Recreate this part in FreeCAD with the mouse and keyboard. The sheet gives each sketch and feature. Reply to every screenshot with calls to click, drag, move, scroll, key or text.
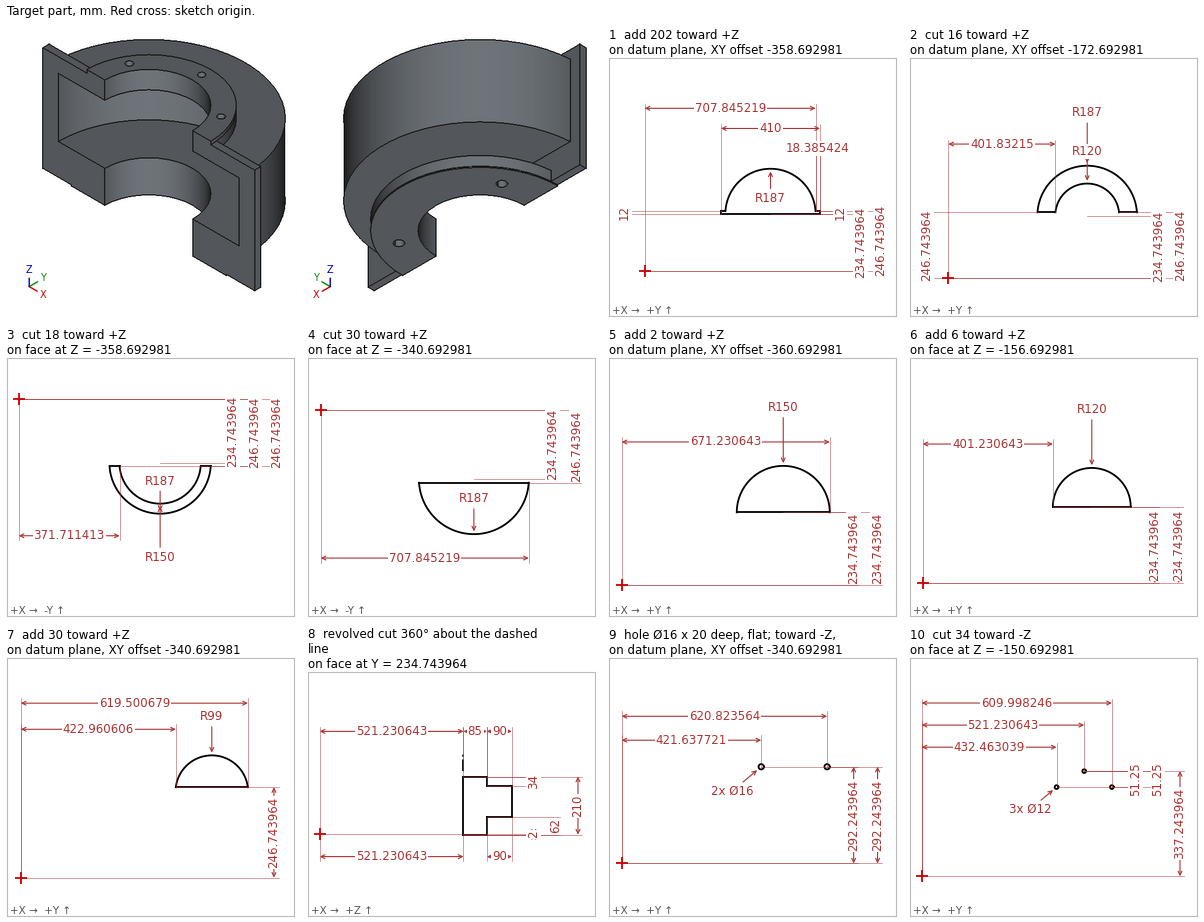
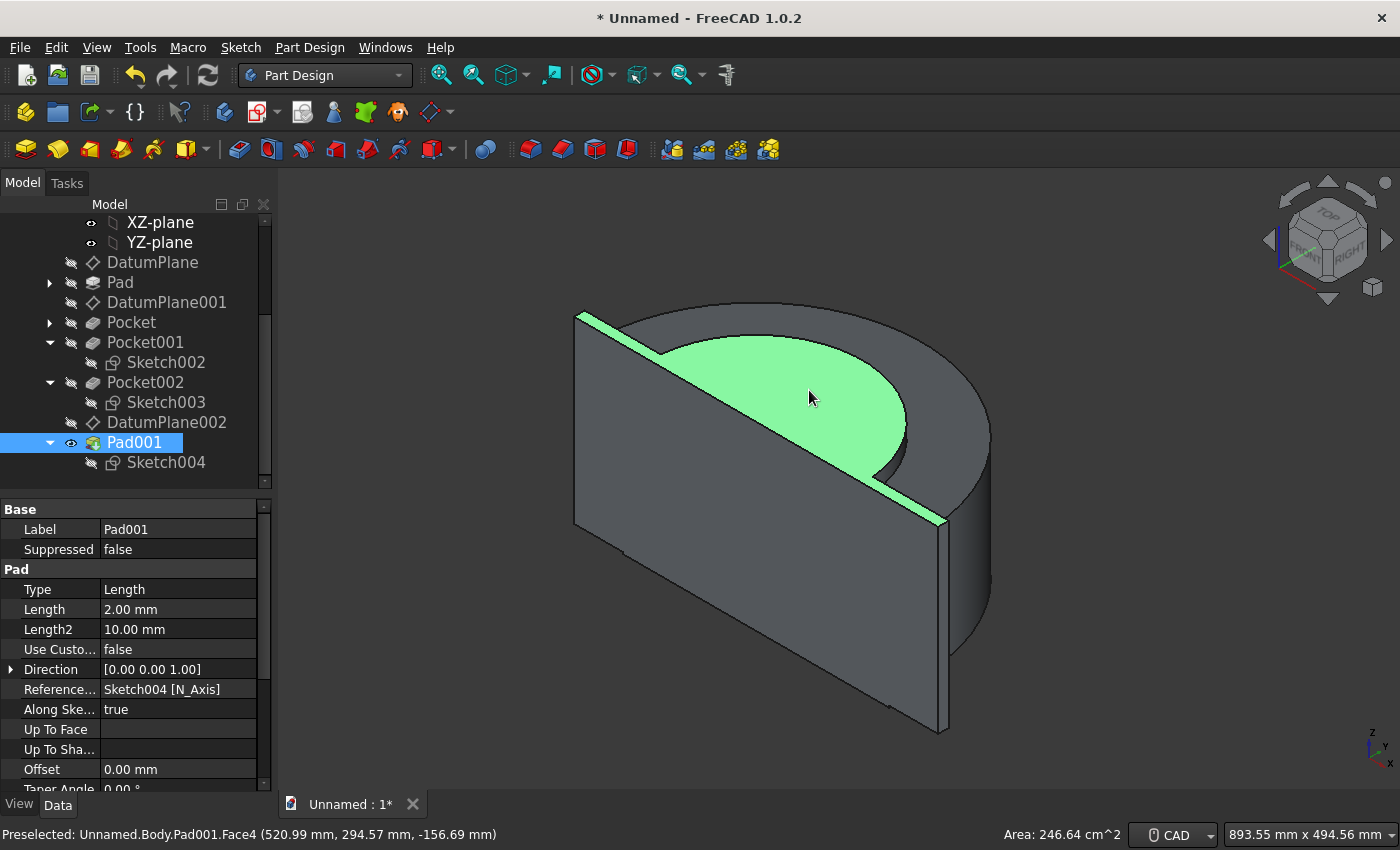
click(258, 112)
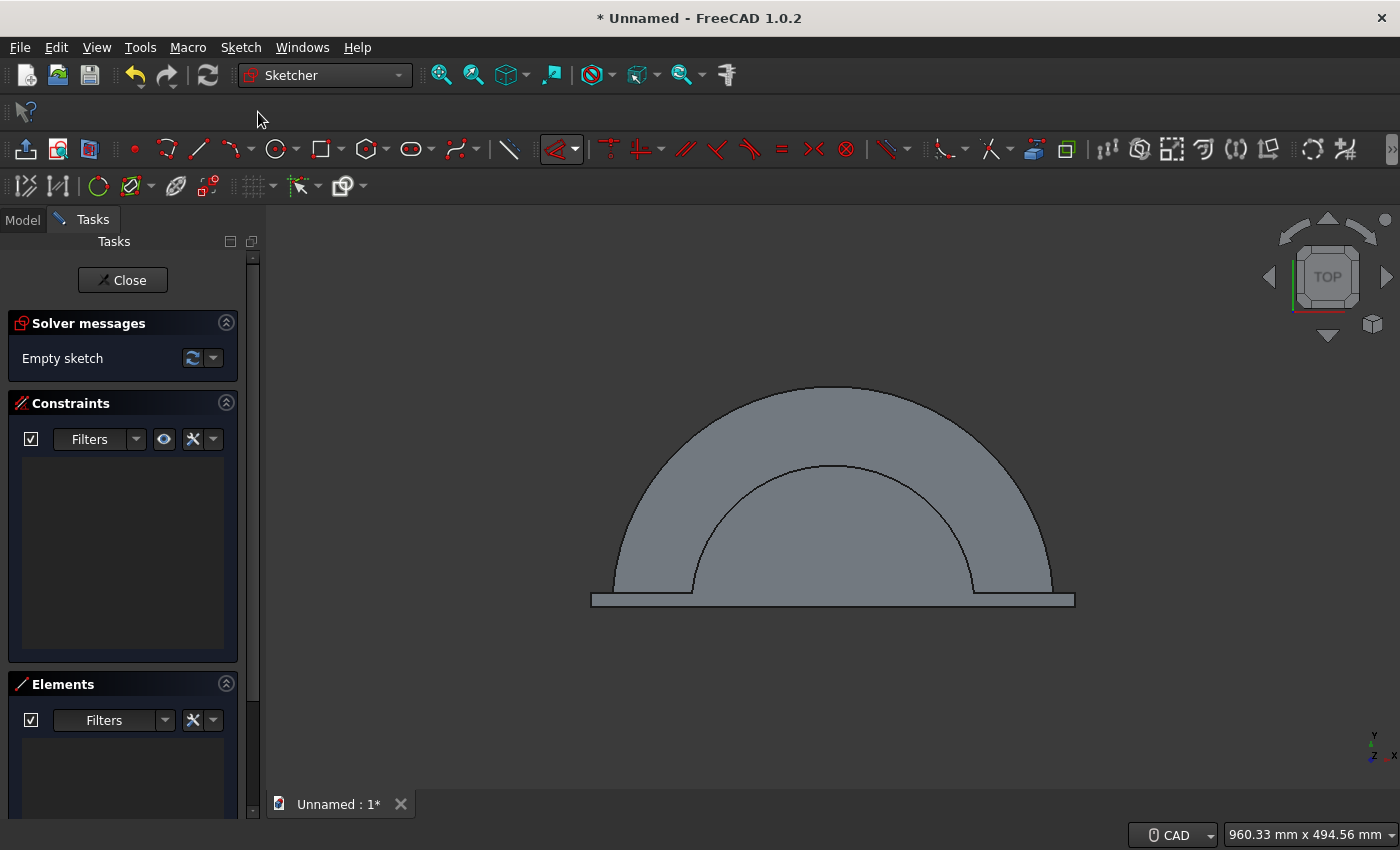
scroll(889, 569, up, 4)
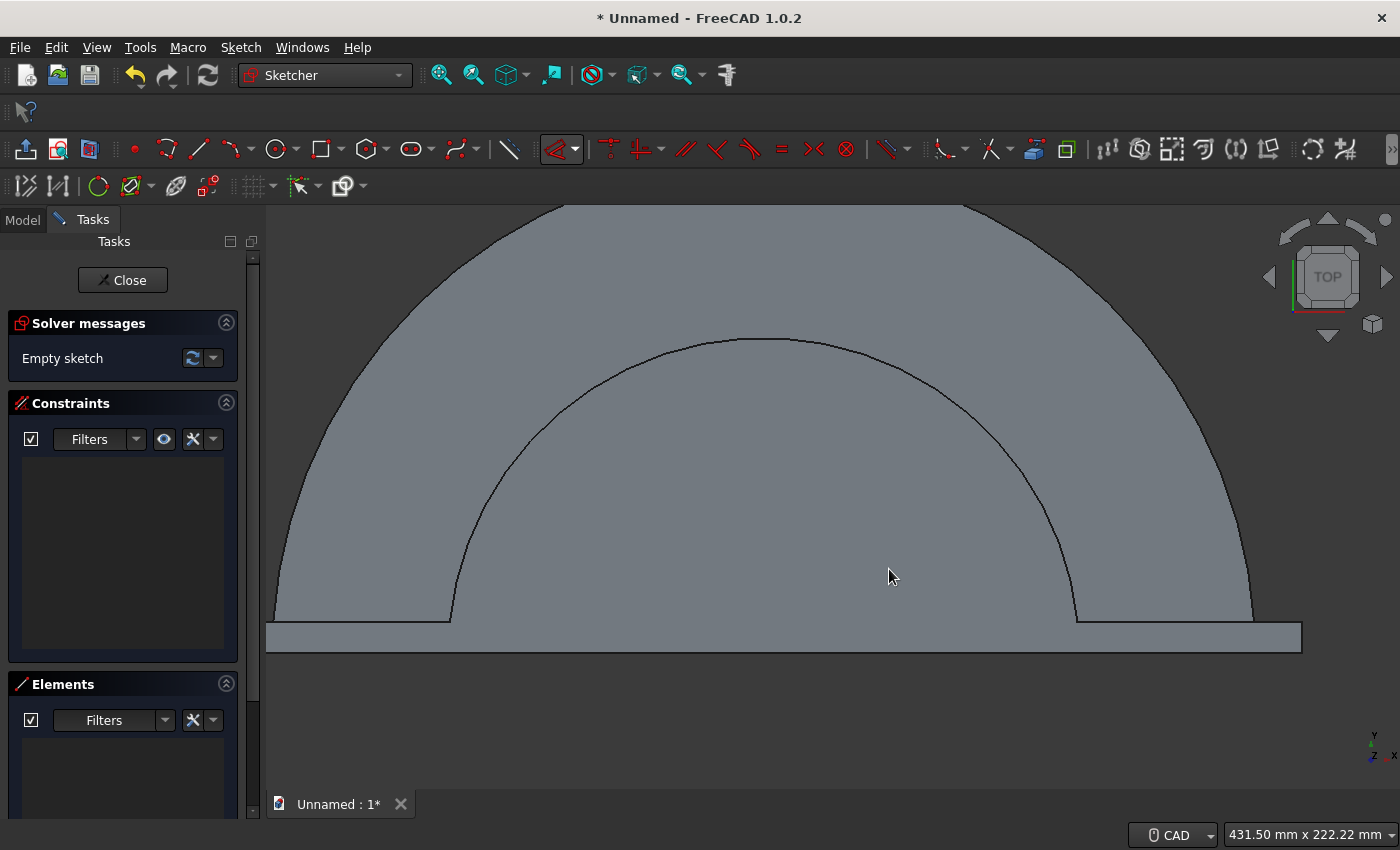
click(200, 150)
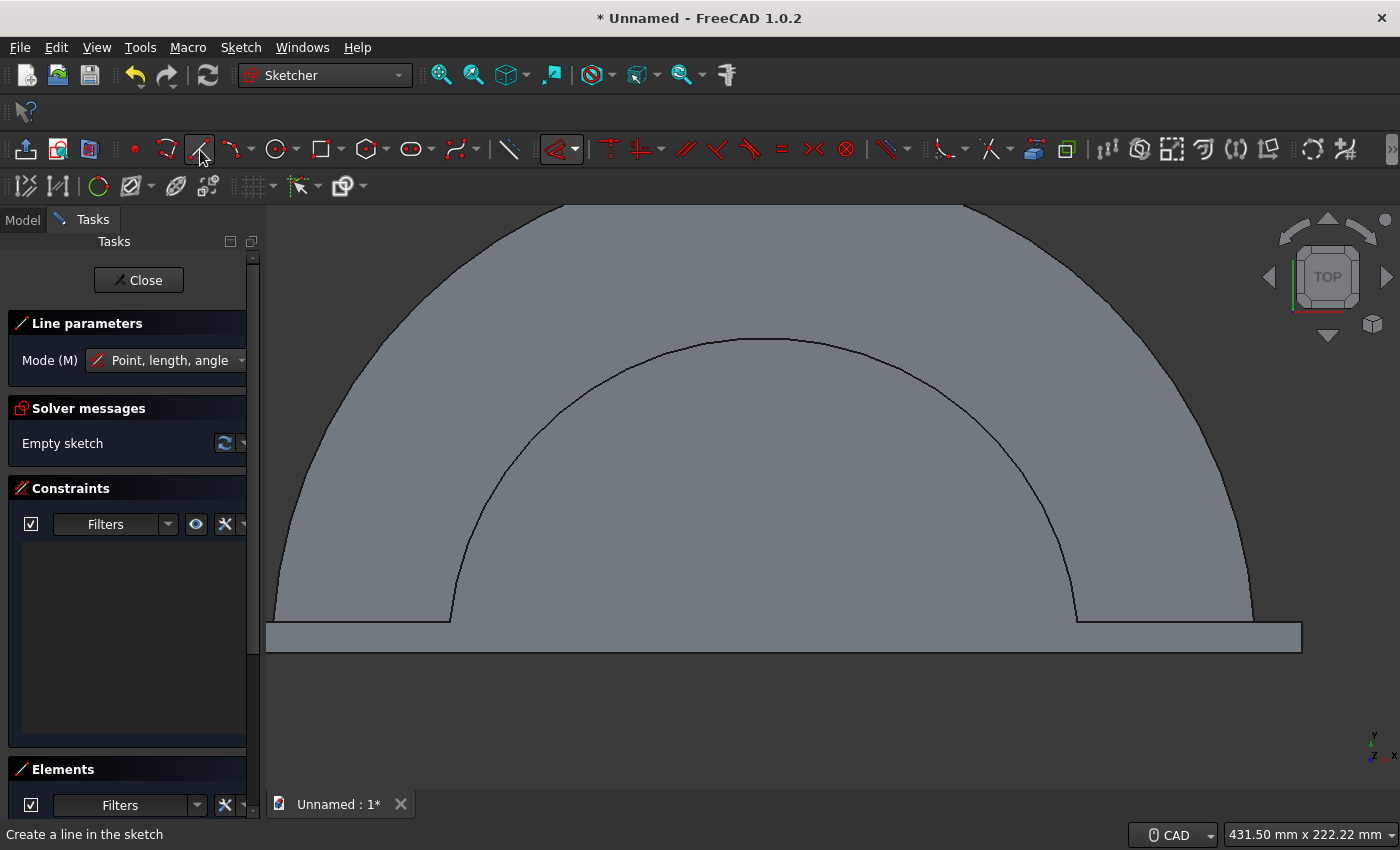
click(448, 653)
click(1079, 653)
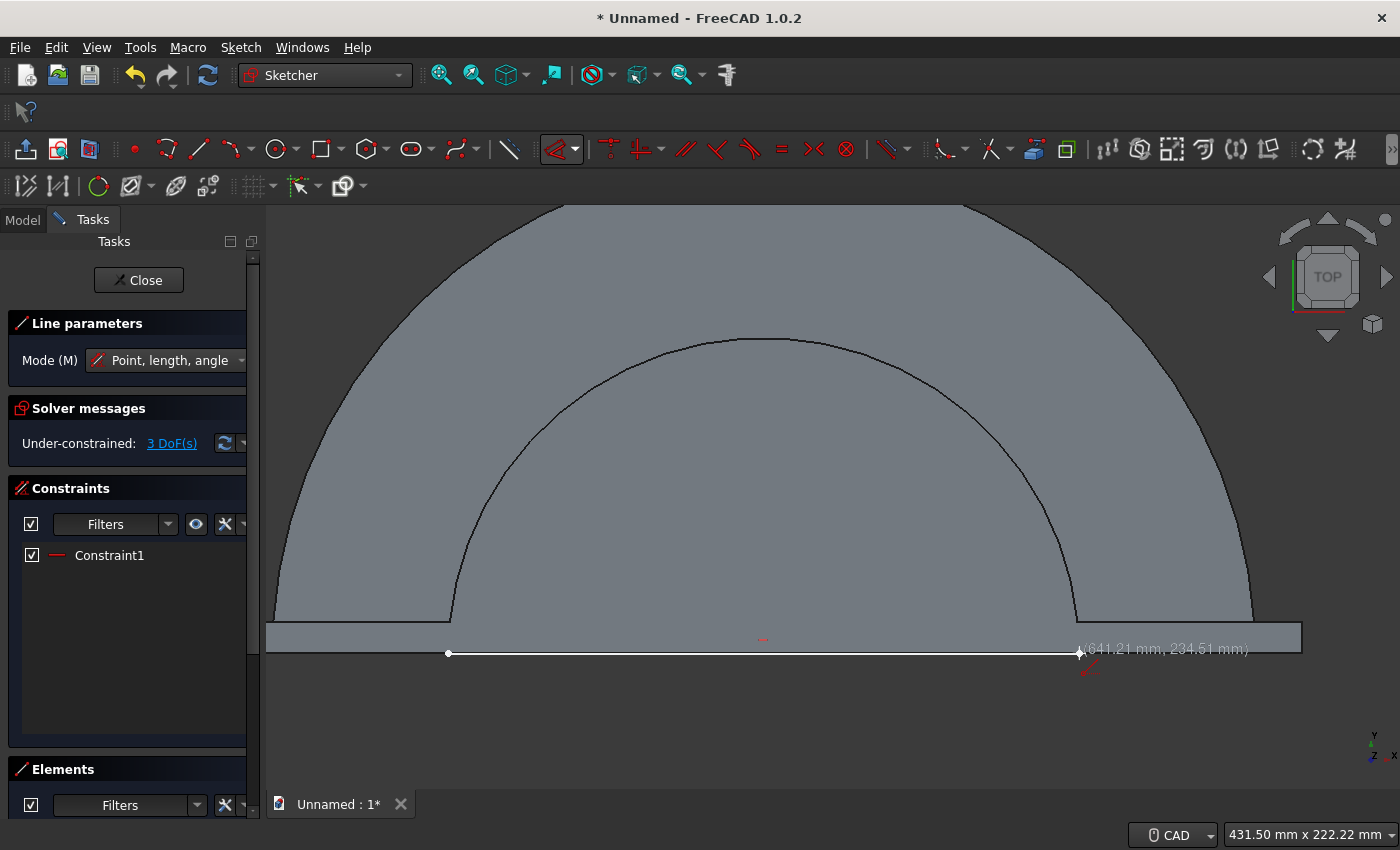
key(g)
key(3)
key(a)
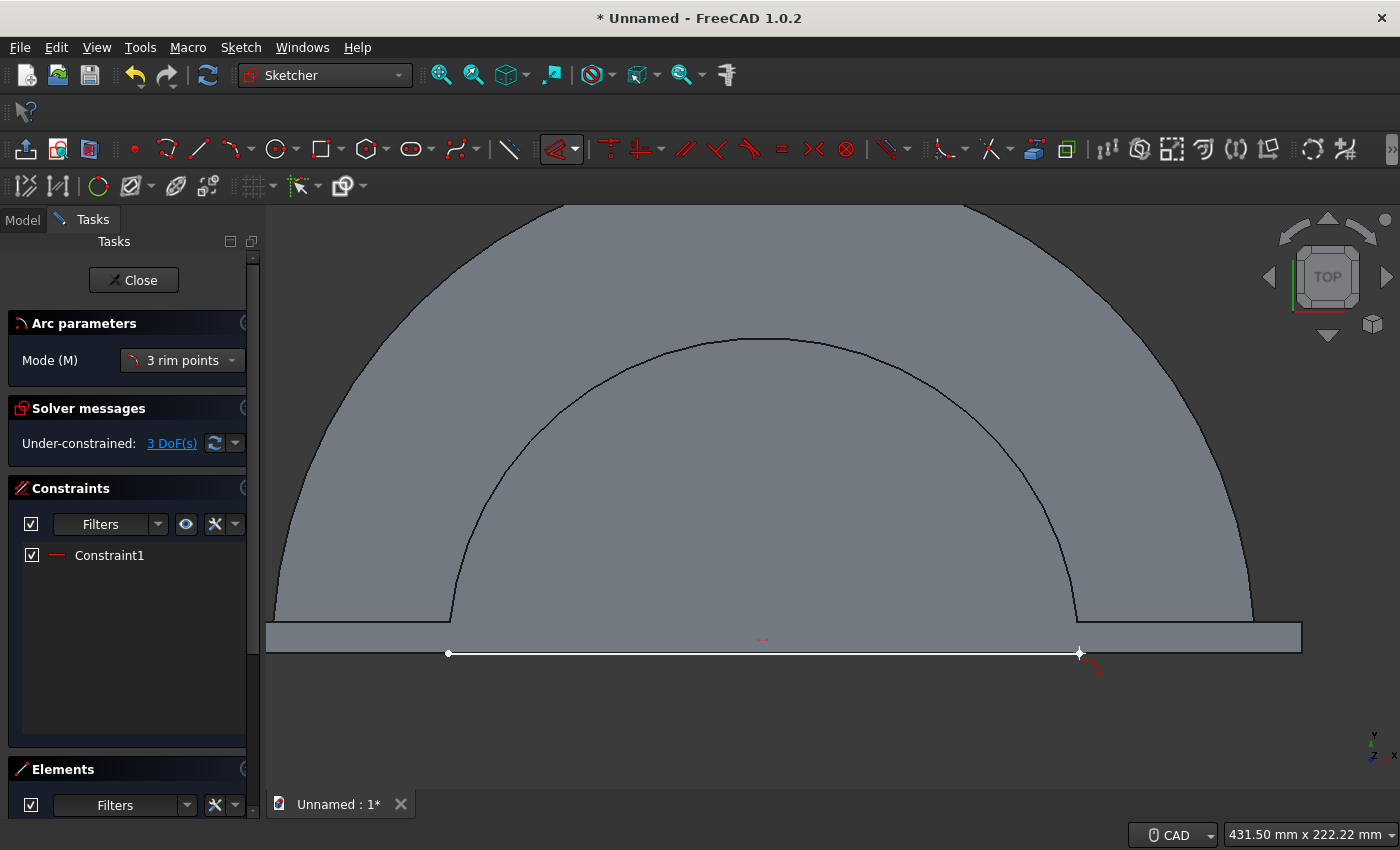
click(1079, 654)
click(448, 654)
click(764, 338)
key(Escape)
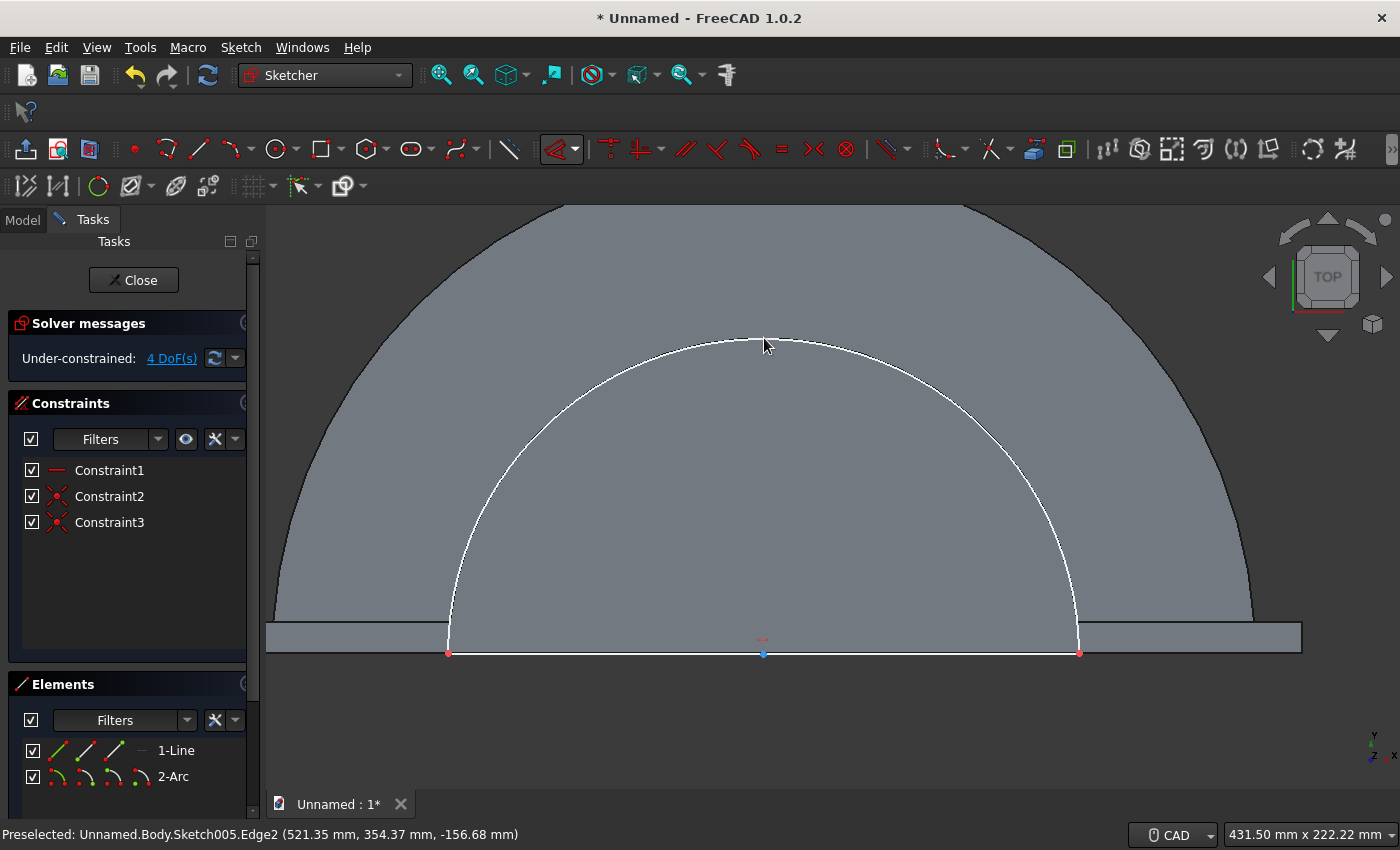
key(d)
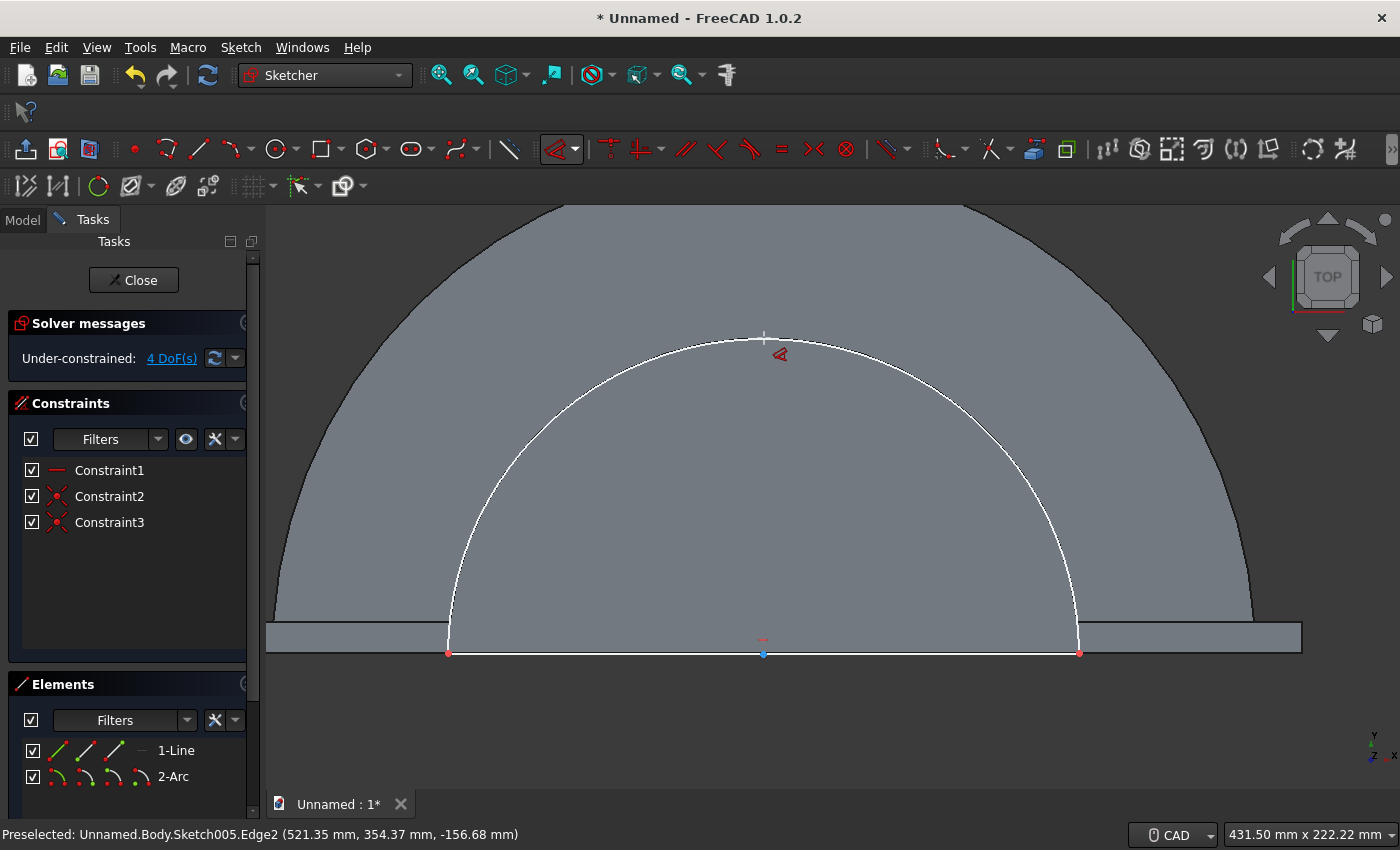
click(949, 399)
click(968, 373)